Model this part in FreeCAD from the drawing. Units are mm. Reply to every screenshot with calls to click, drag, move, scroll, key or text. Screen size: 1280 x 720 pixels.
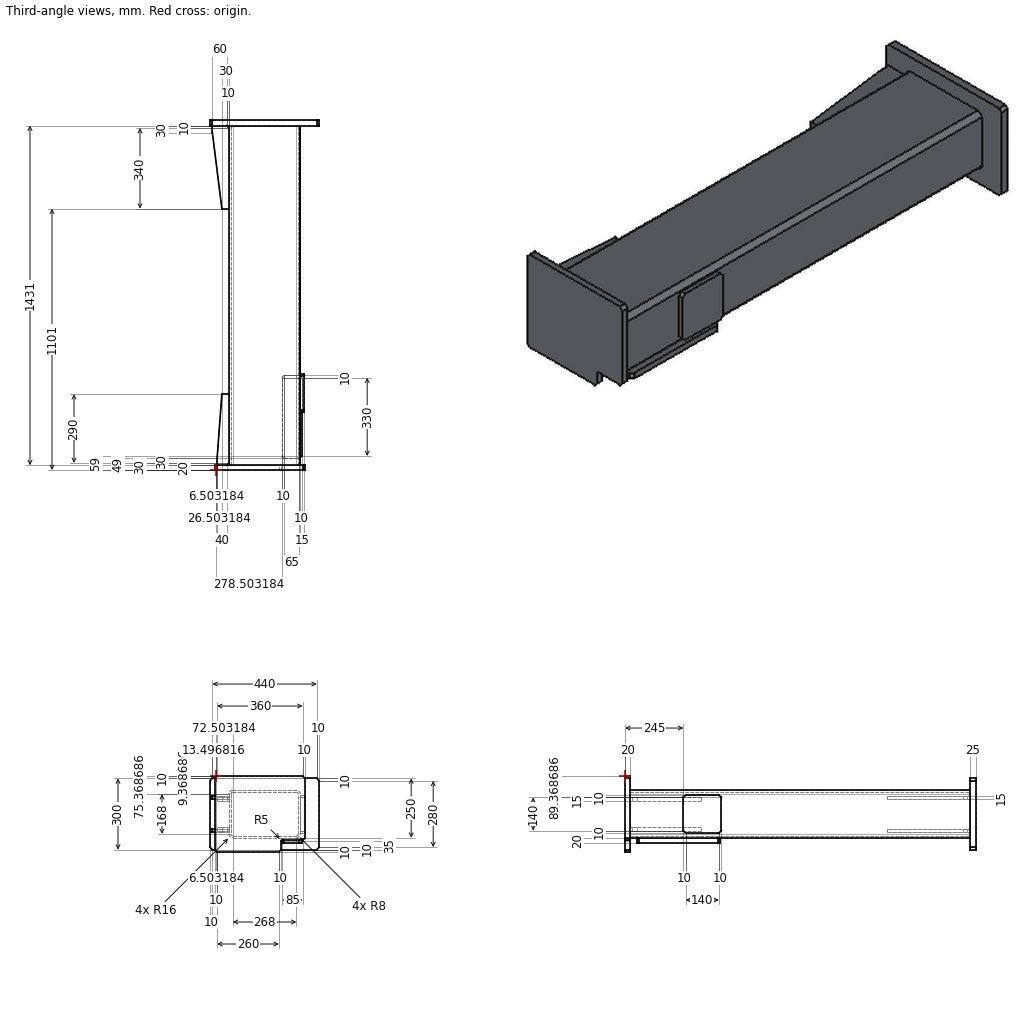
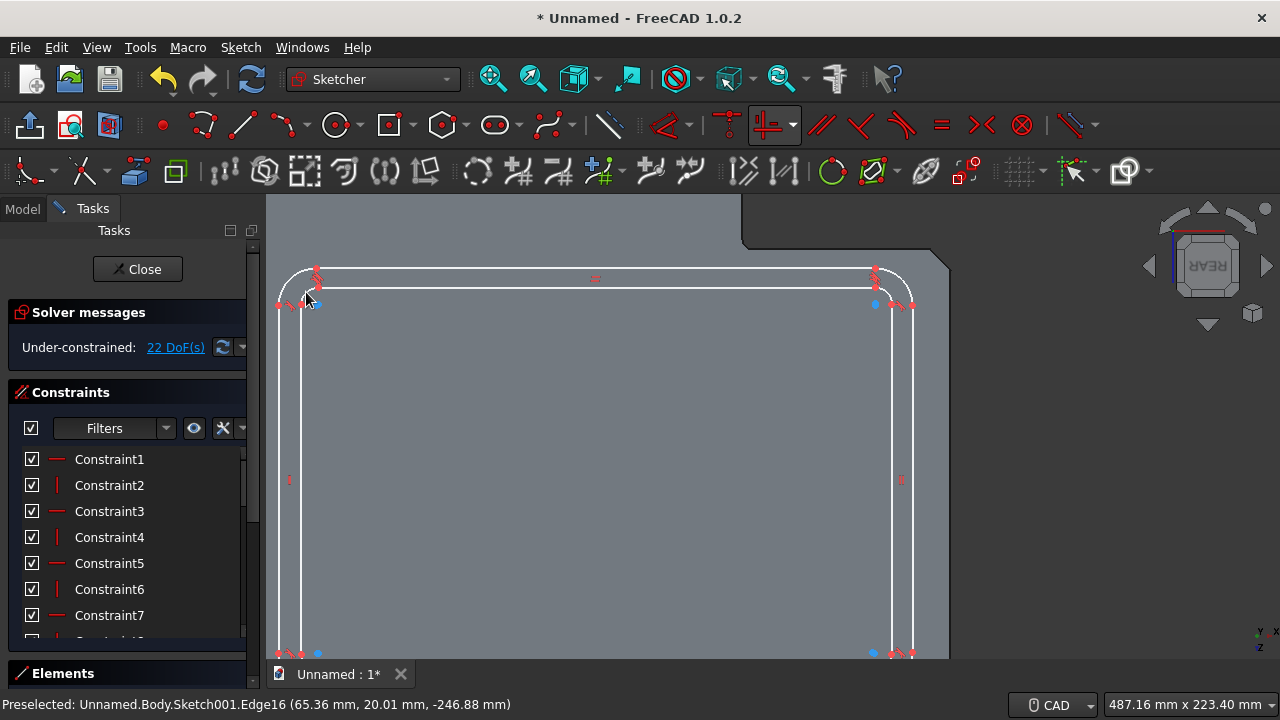
click(892, 409)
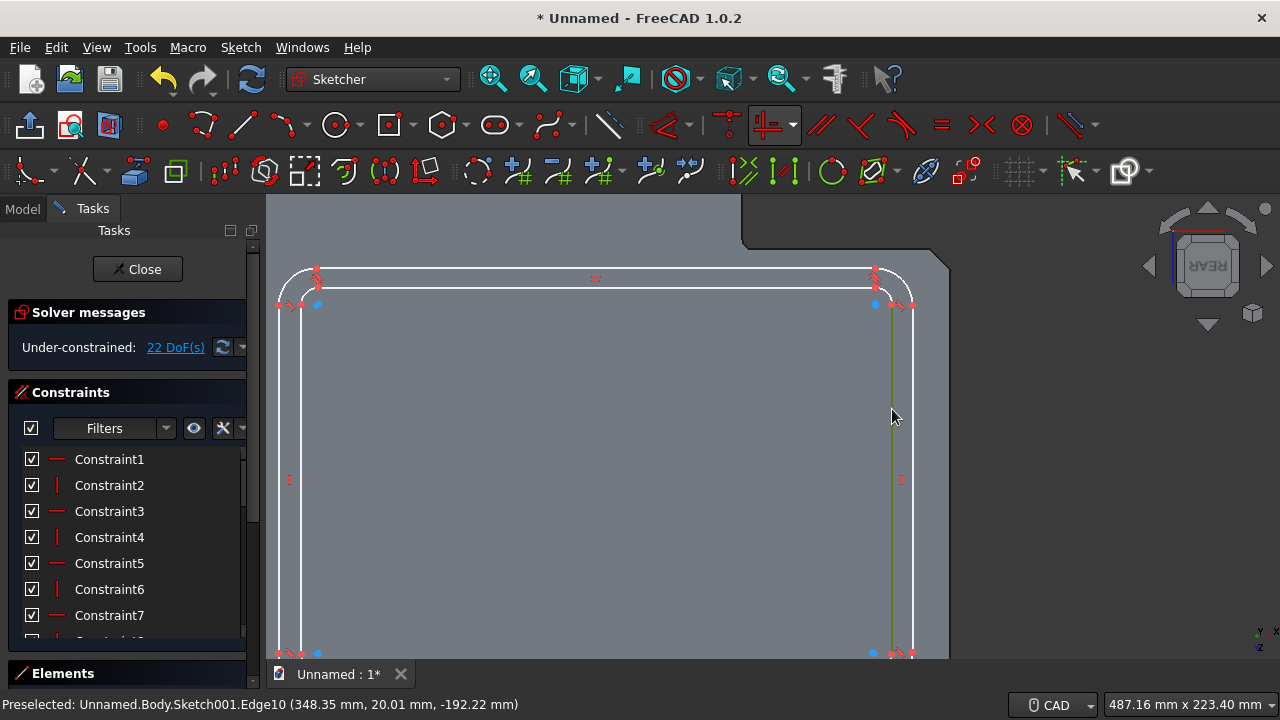
click(887, 293)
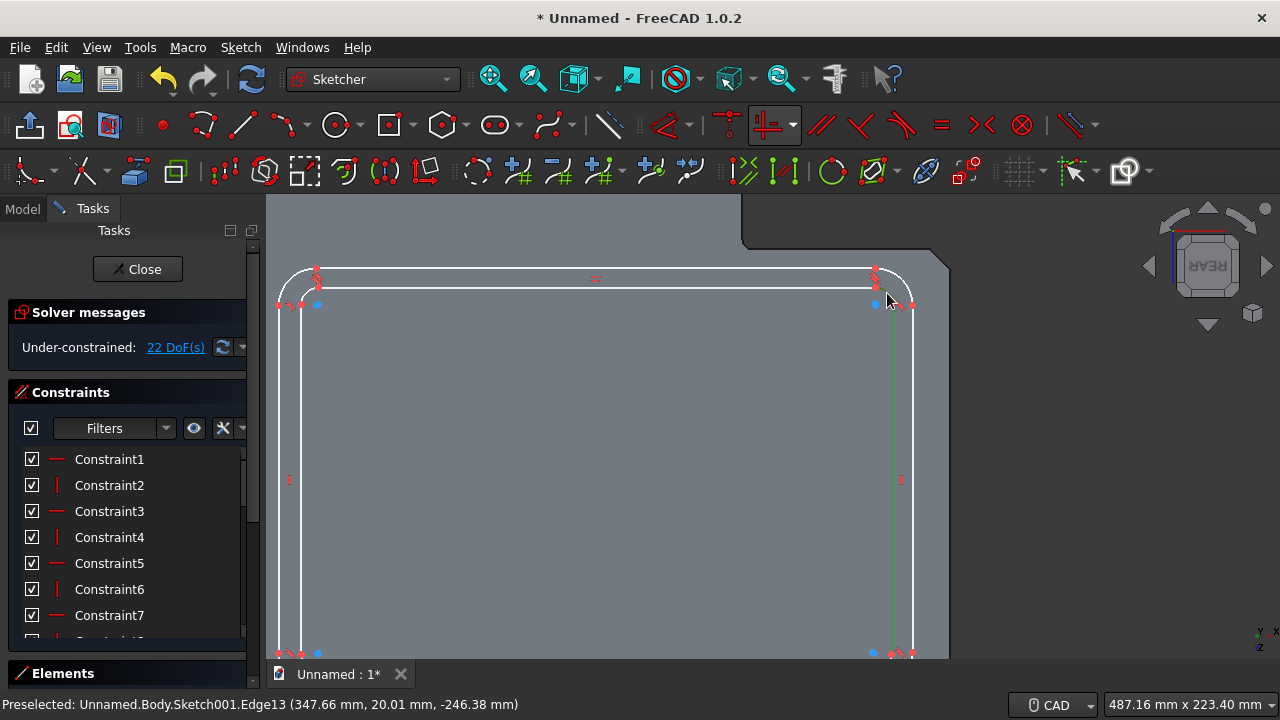
click(902, 126)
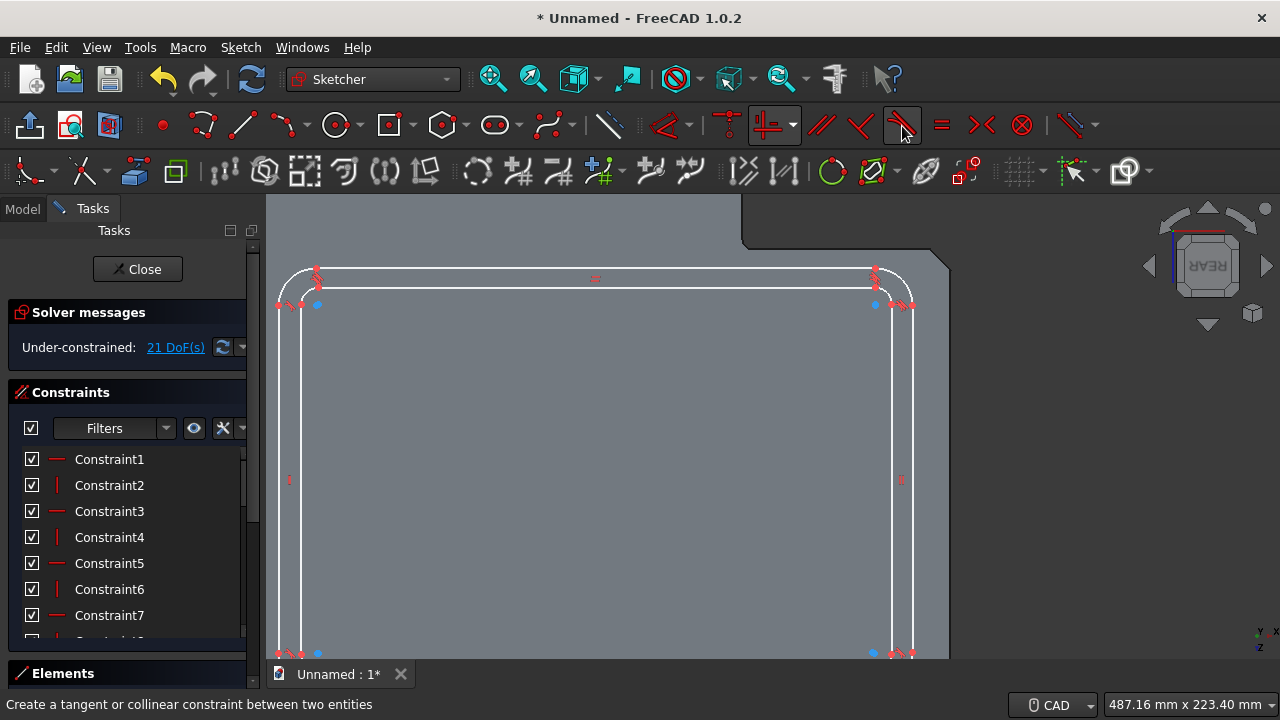
click(892, 409)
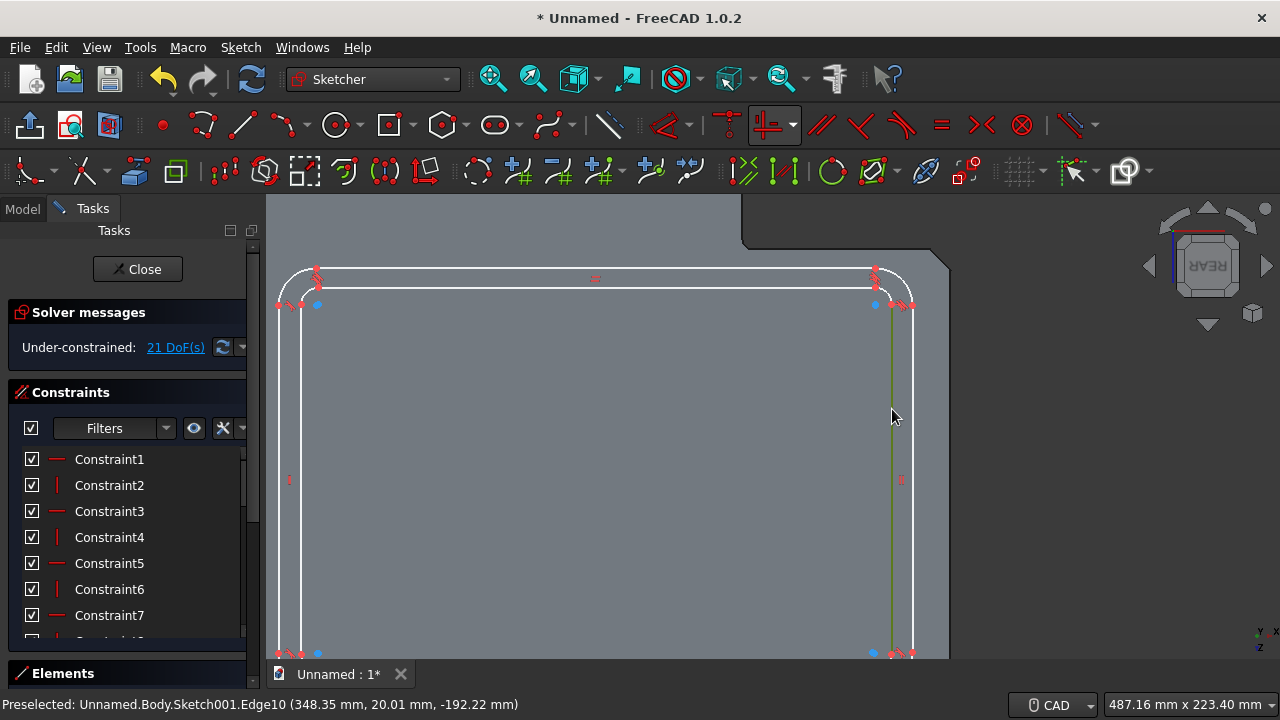
scroll(907, 288, down, 3)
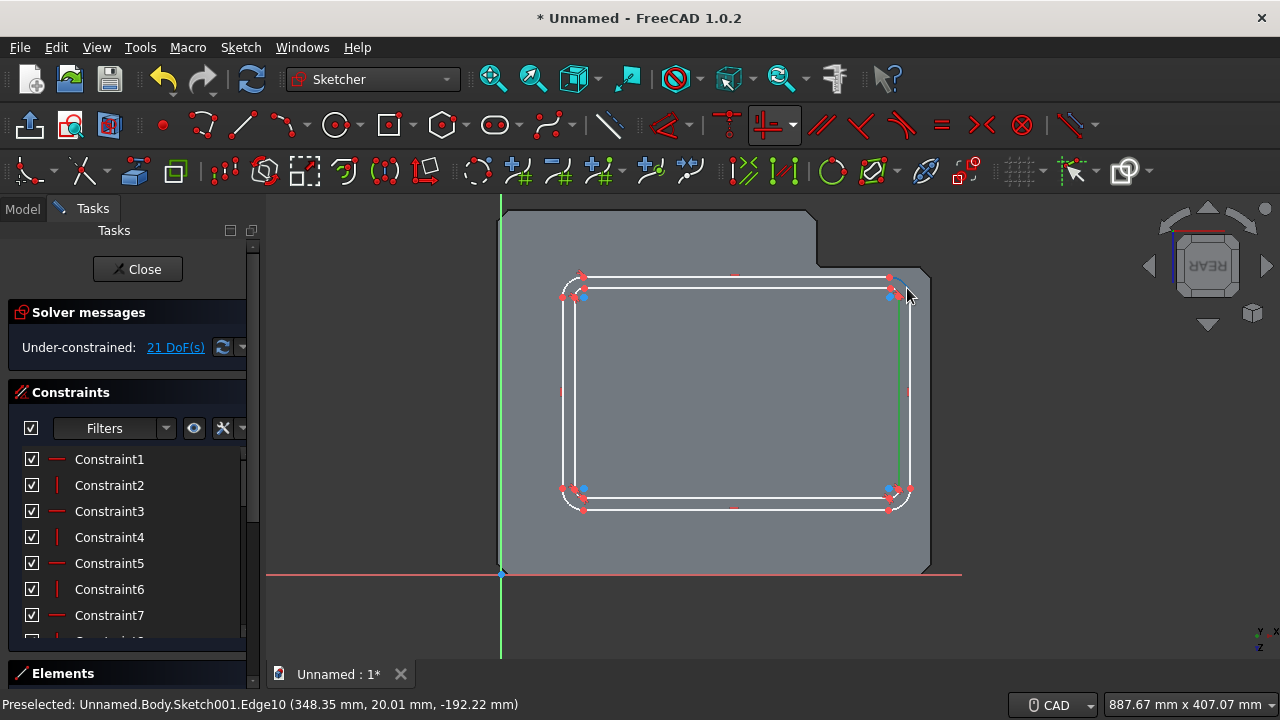
scroll(896, 495, up, 4)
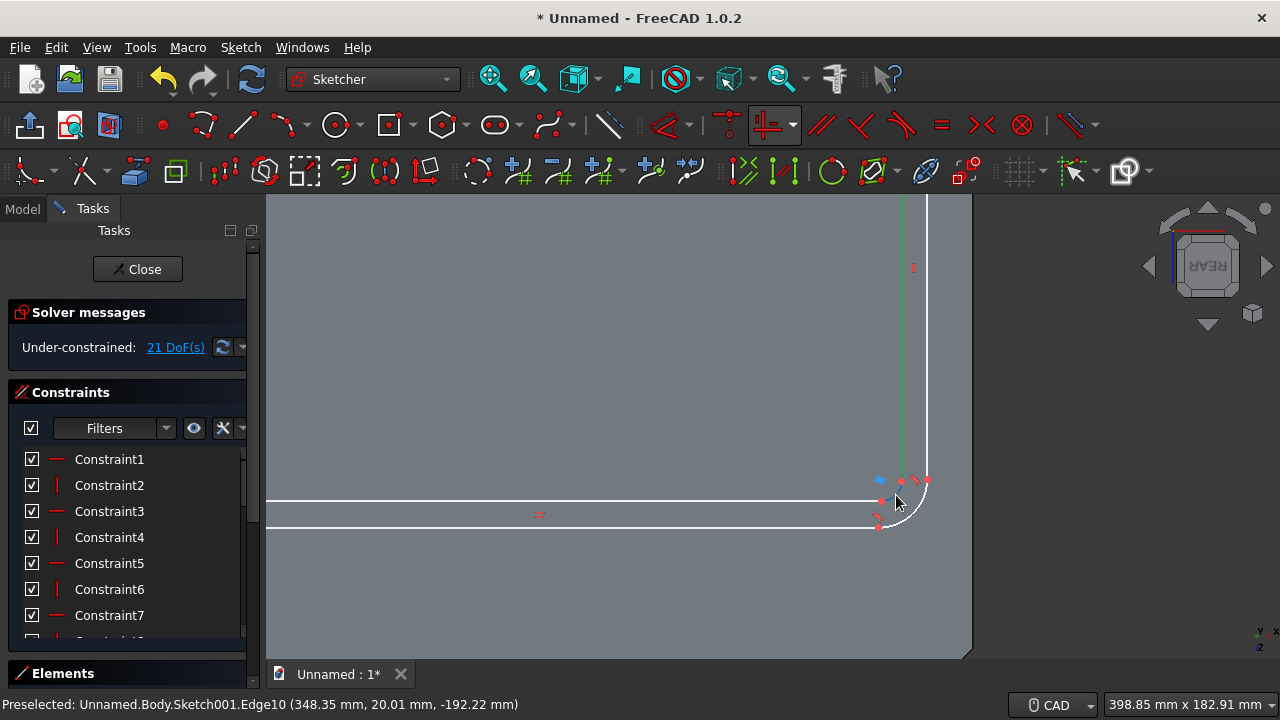
click(896, 495)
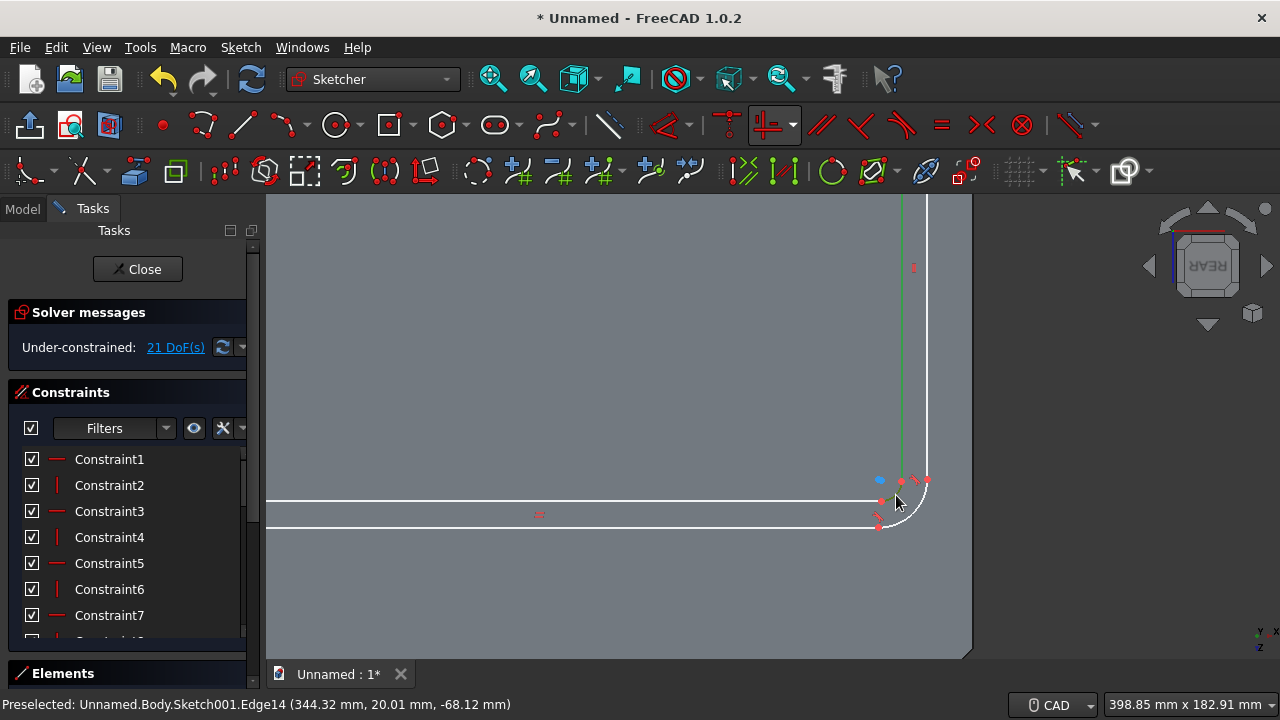
click(902, 126)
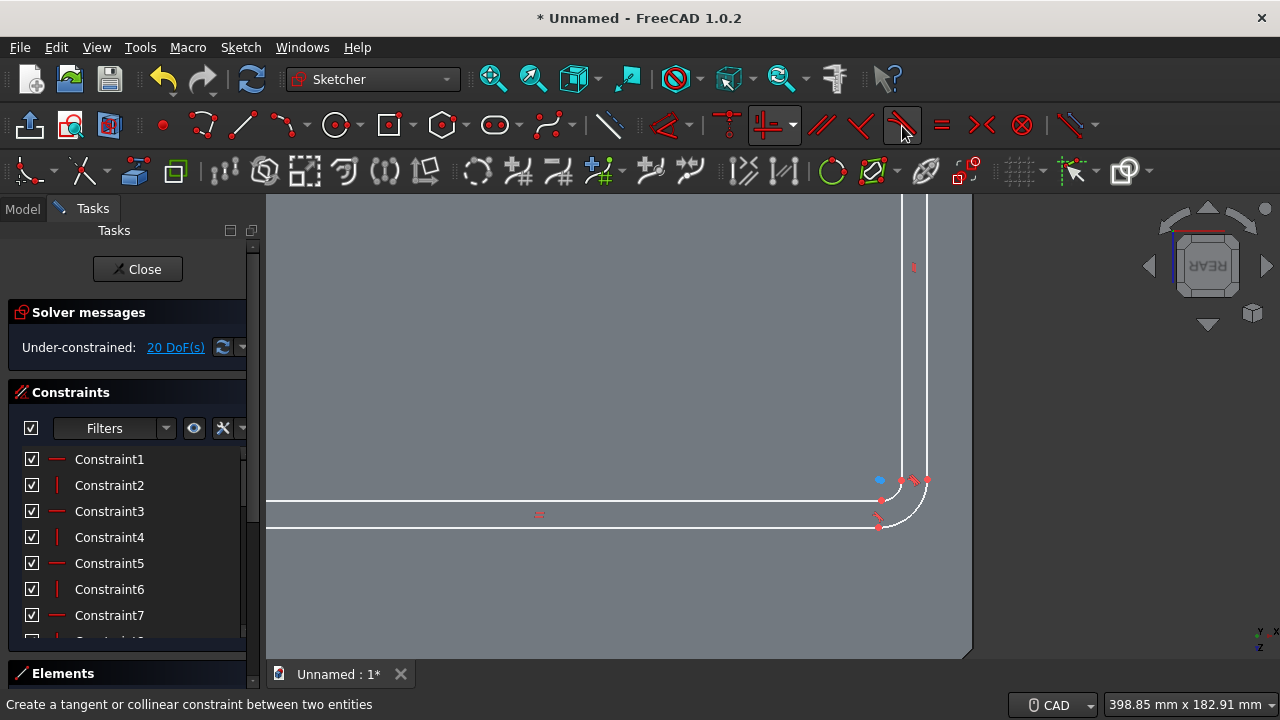
click(677, 501)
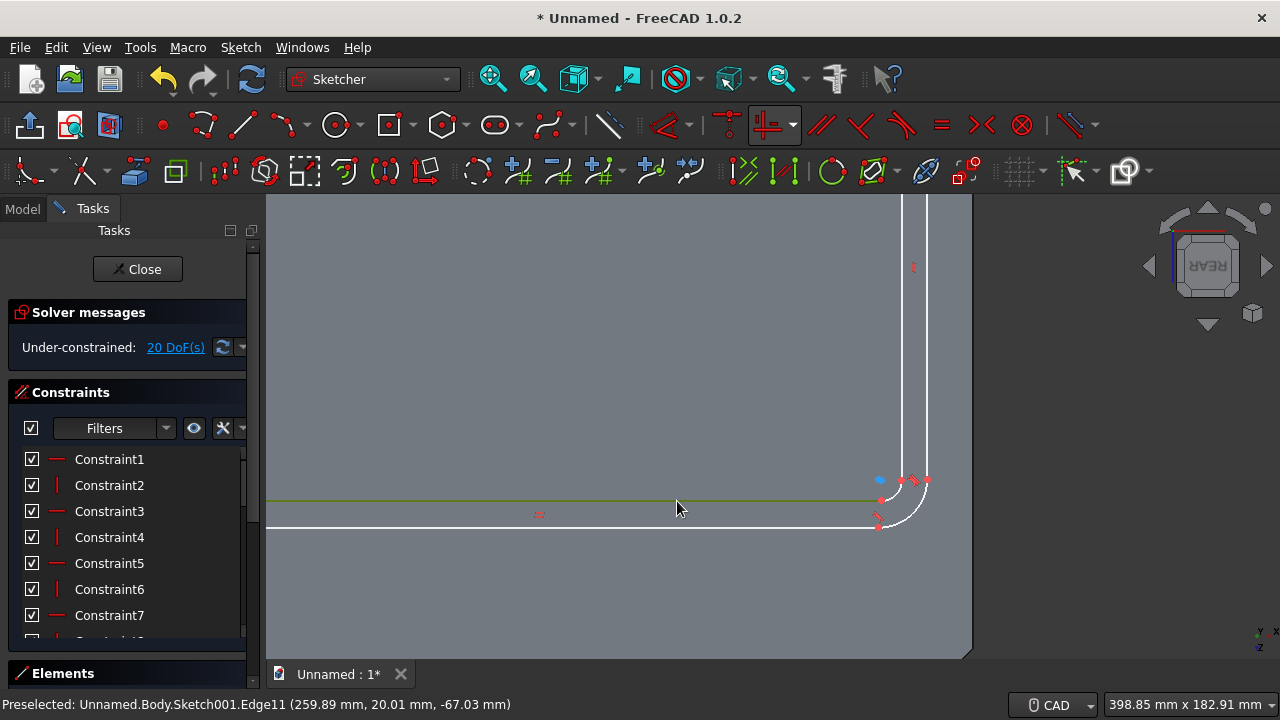
scroll(891, 499, up, 2)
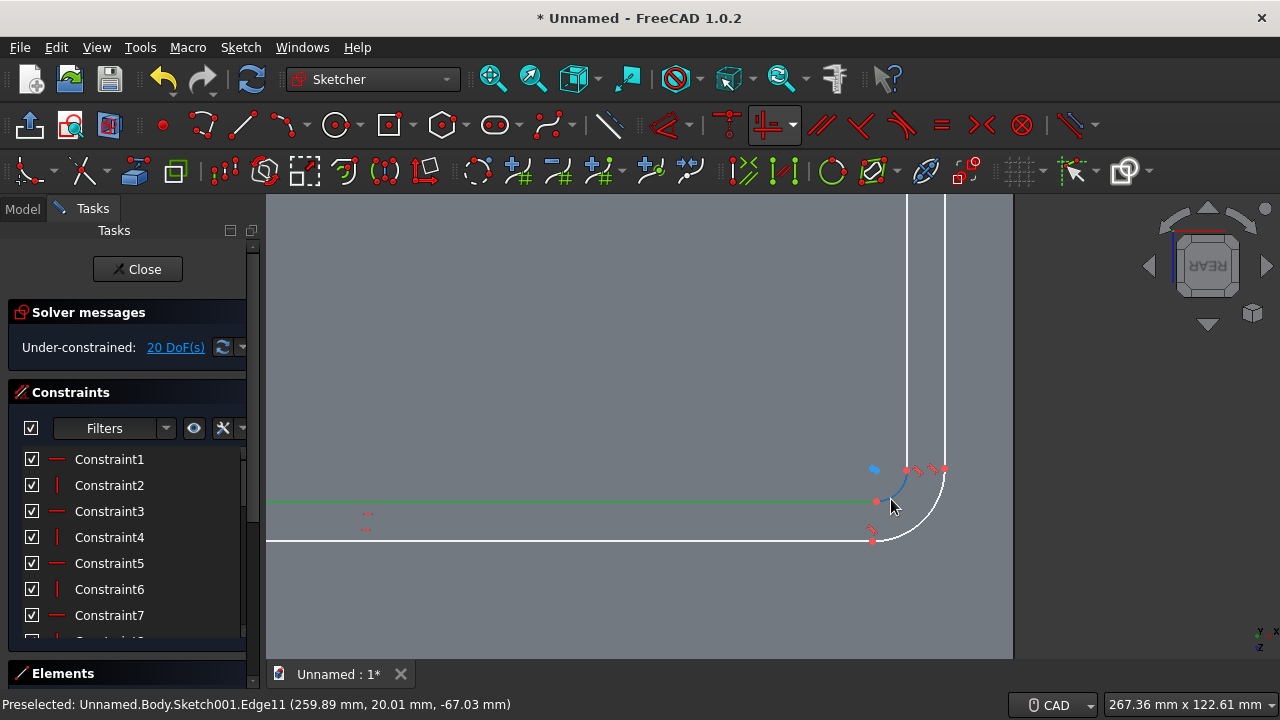
click(890, 498)